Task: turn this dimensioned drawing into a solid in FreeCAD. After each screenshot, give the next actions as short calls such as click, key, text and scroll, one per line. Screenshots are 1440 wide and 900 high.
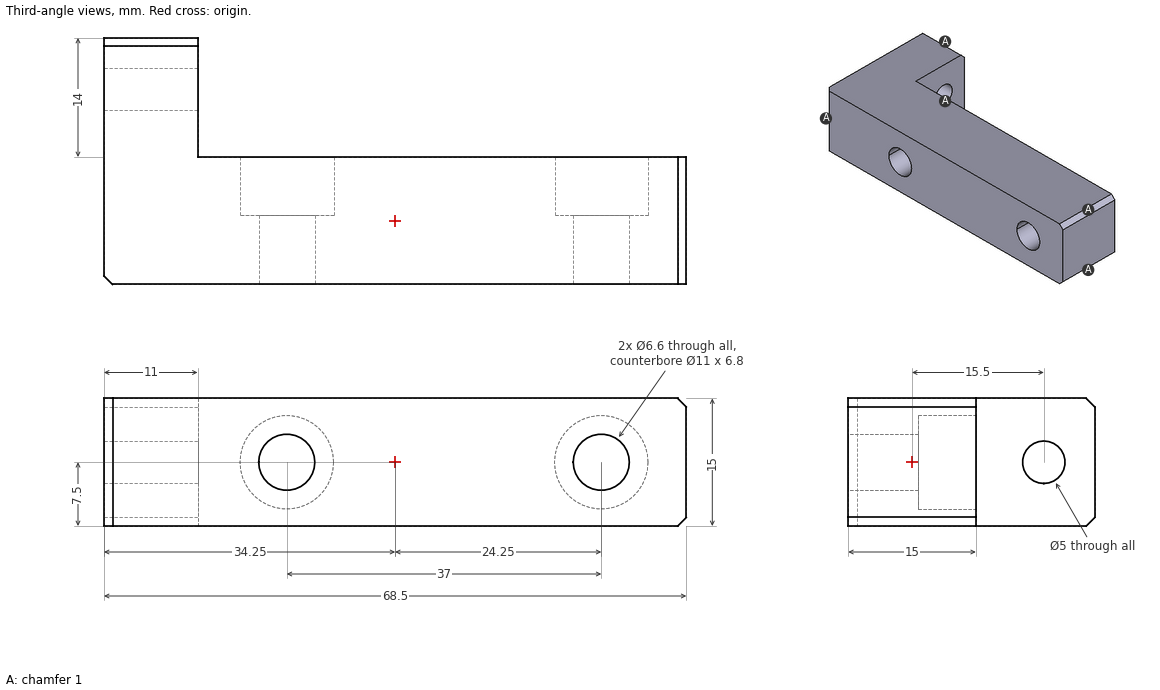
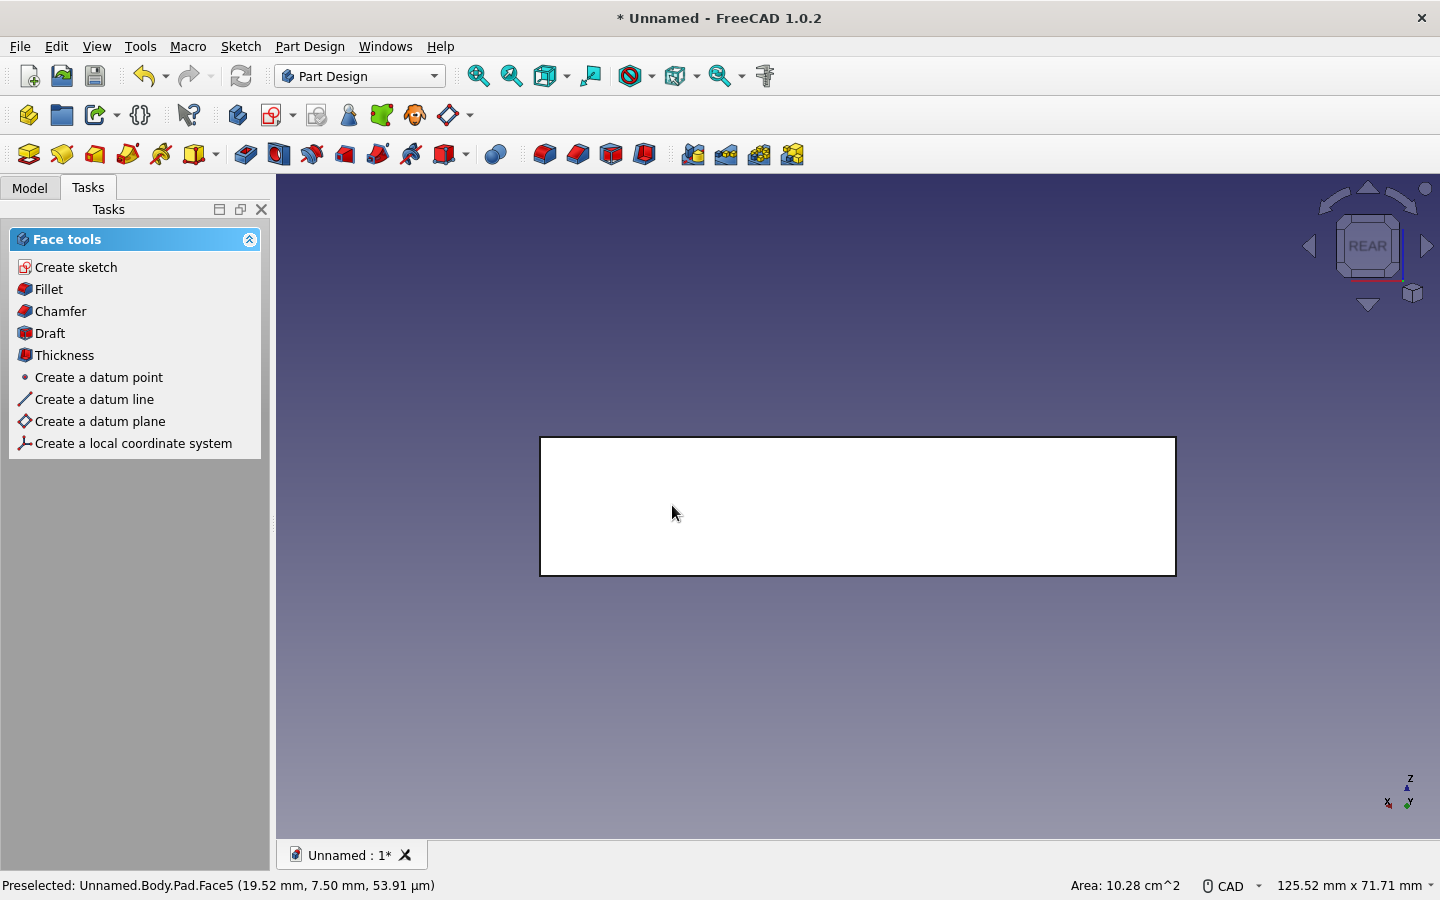
click(270, 116)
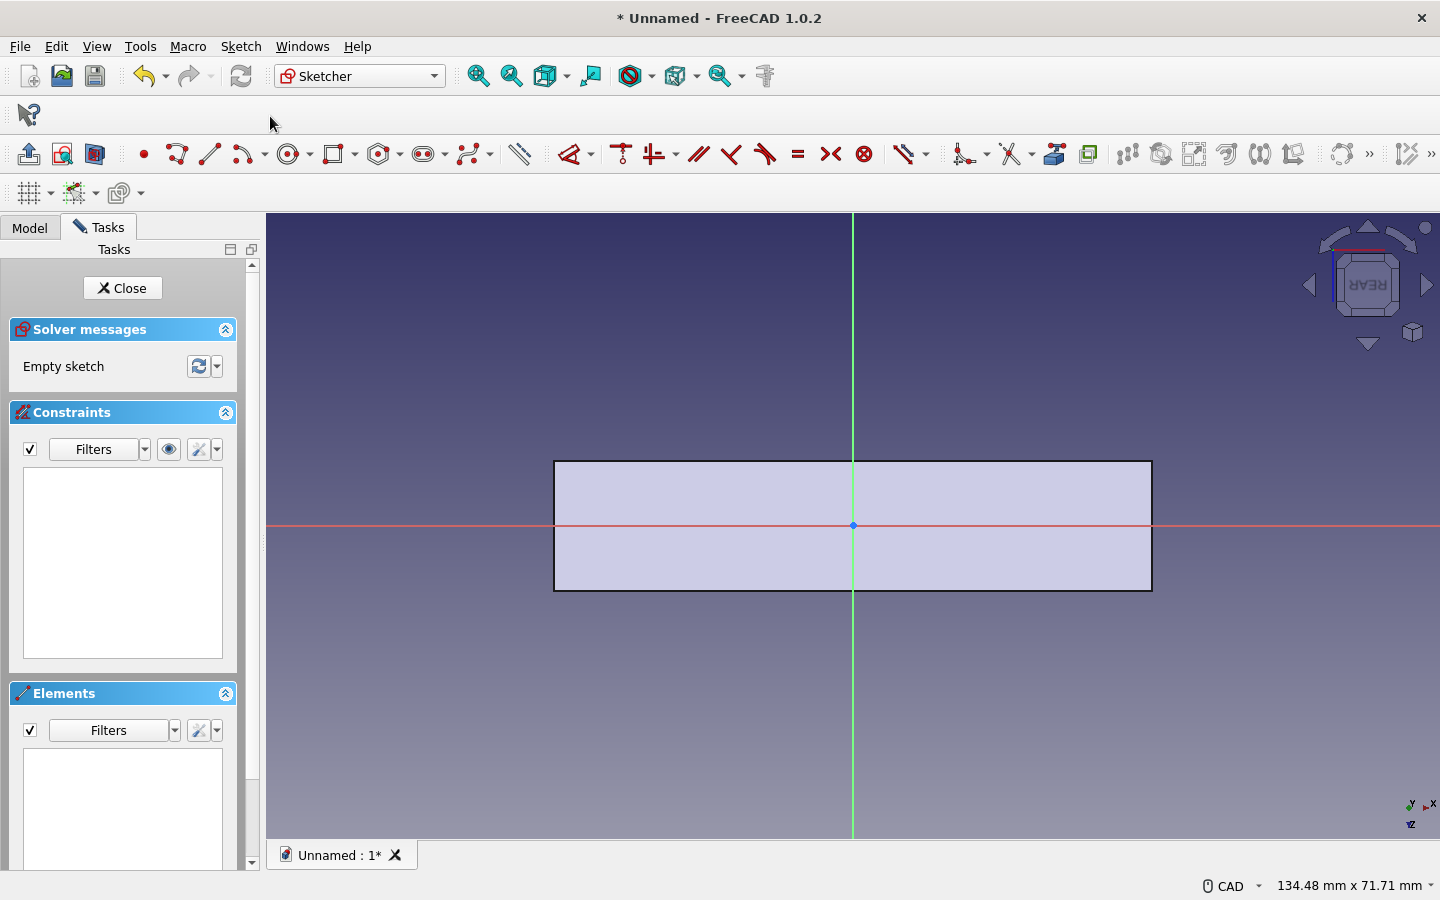
scroll(637, 526, up, 4)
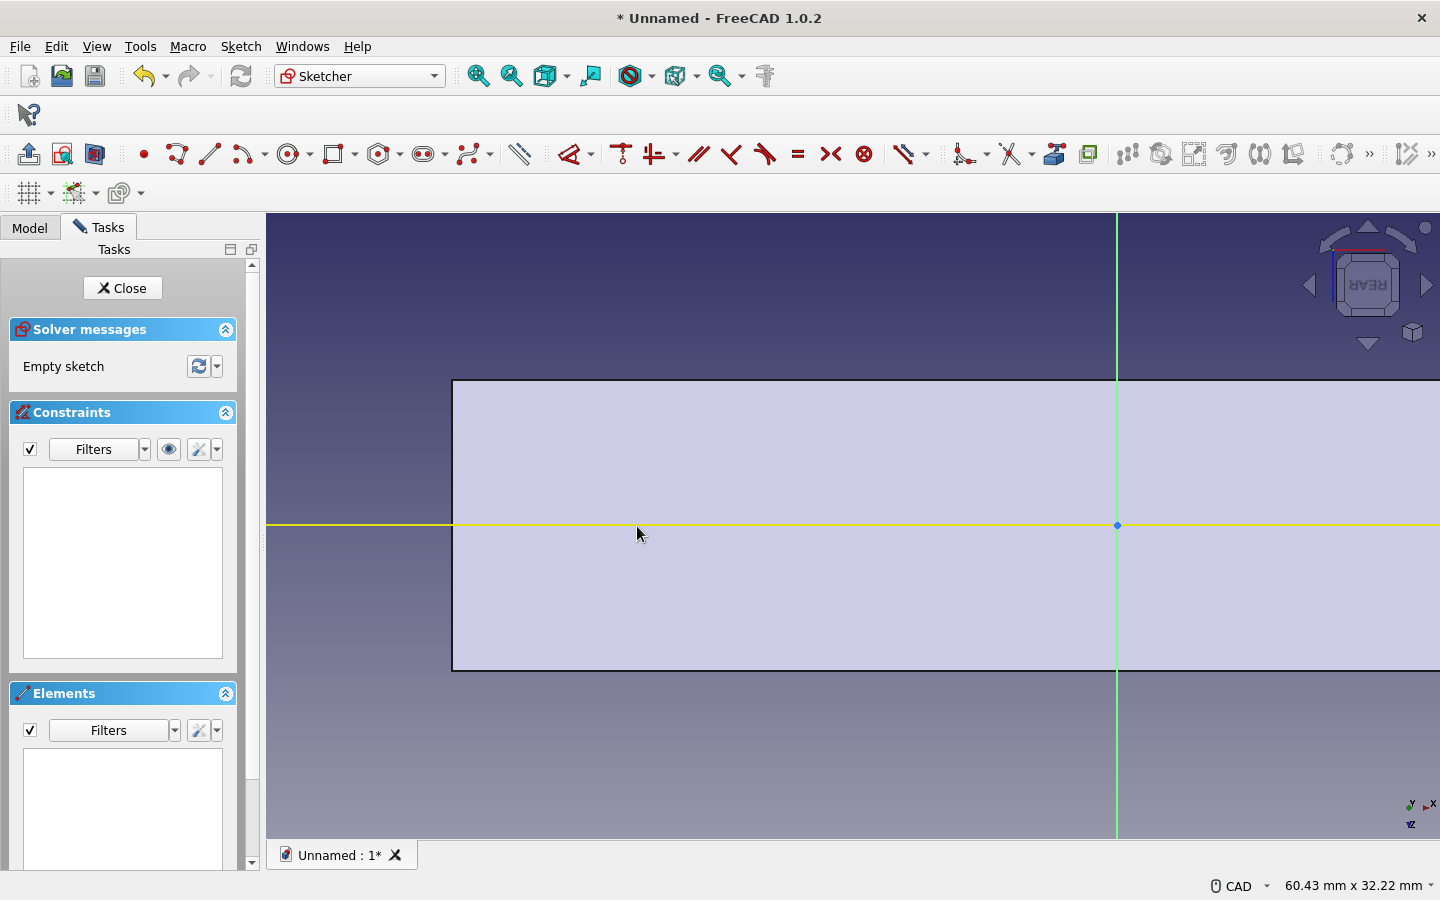
click(332, 154)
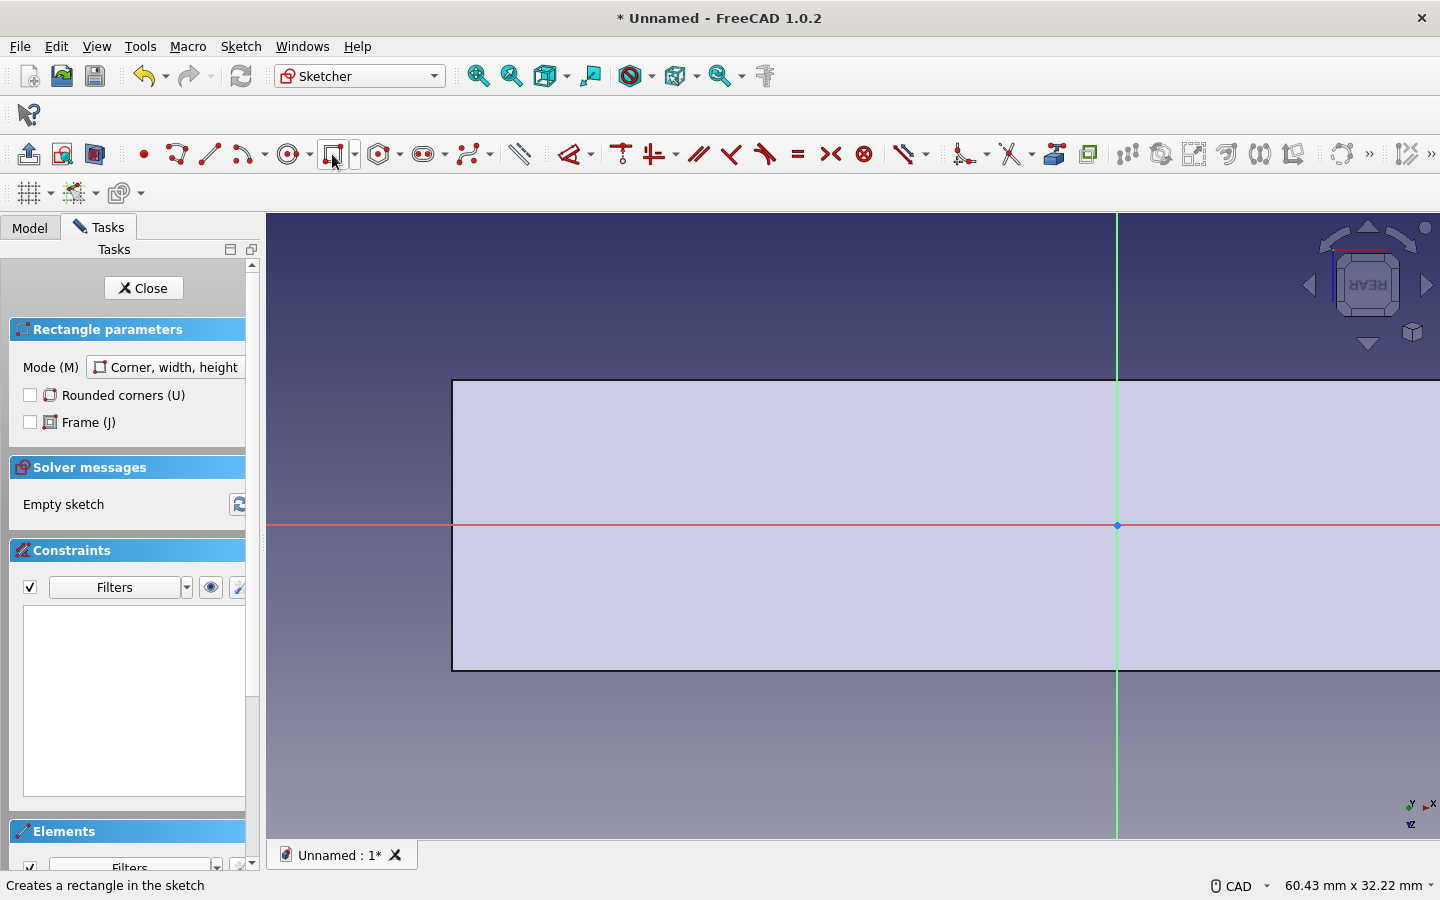
click(452, 380)
move(666, 671)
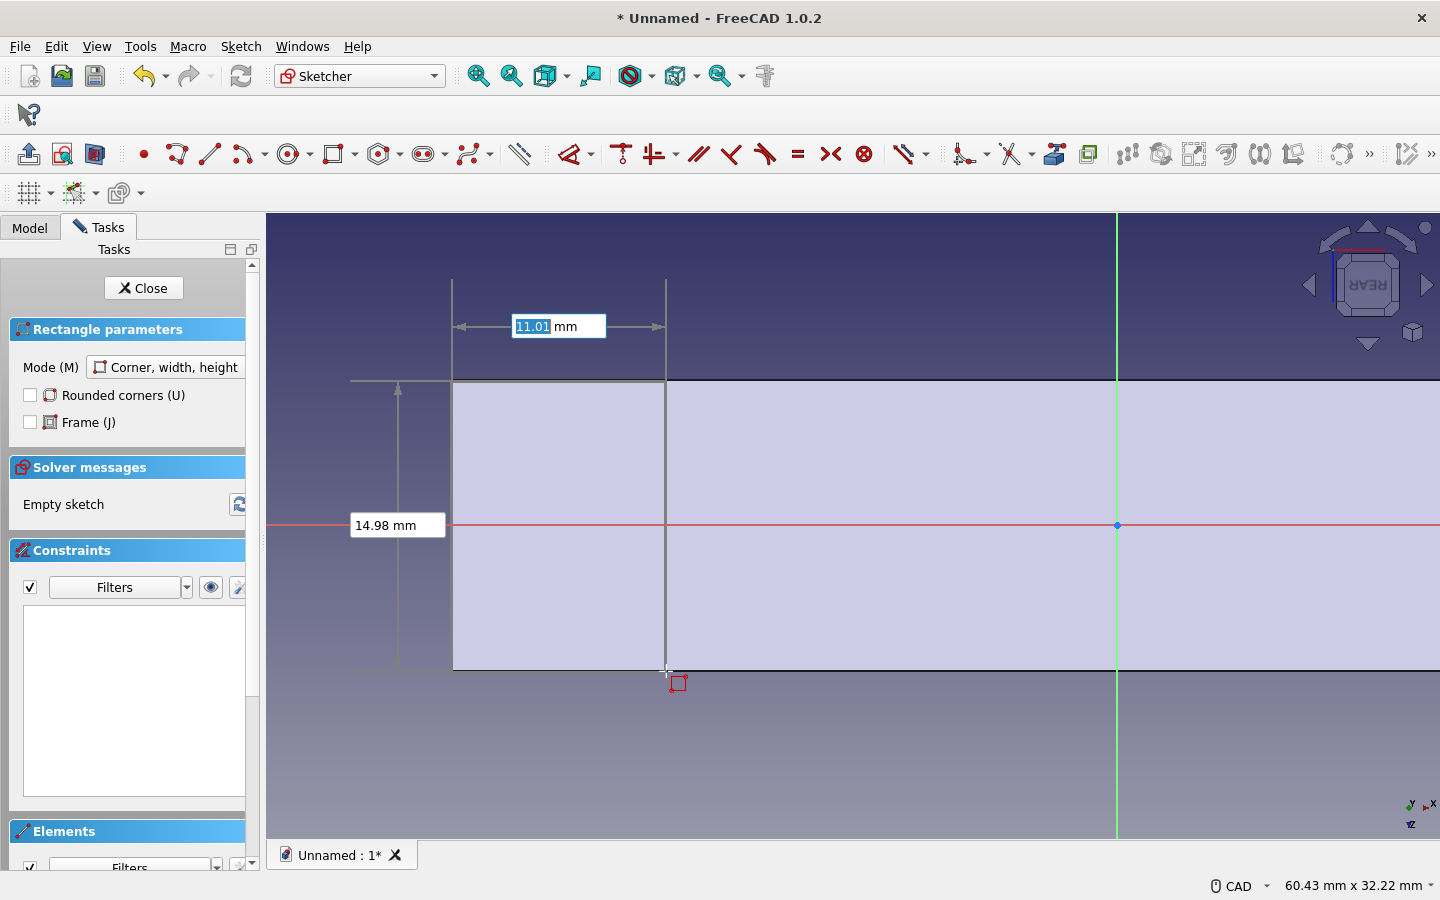
text(11)
key(Tab)
text(15)
key(Return)
key(Escape)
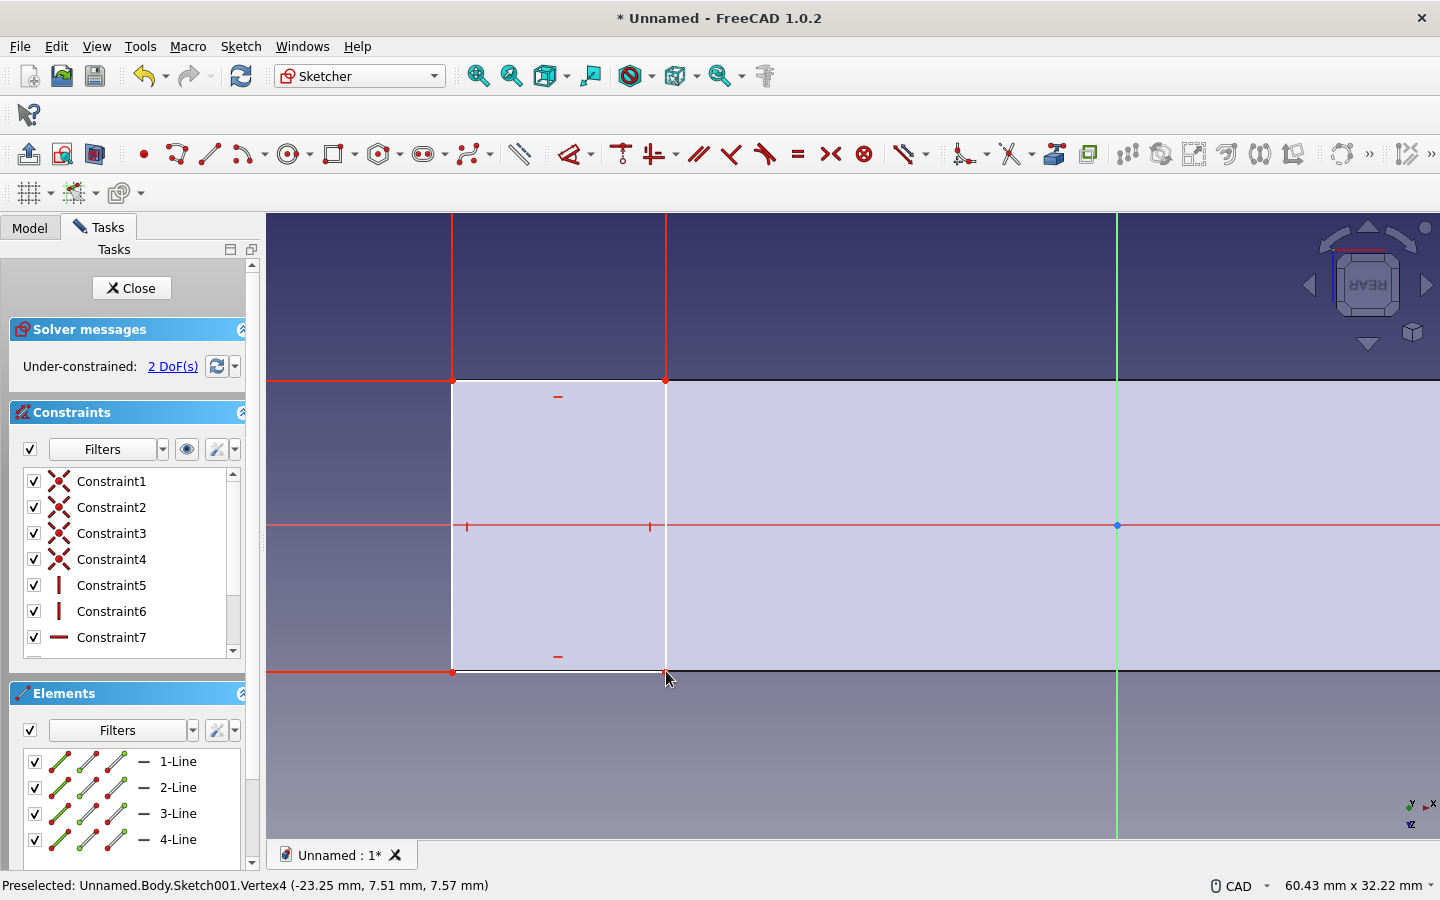
click(568, 154)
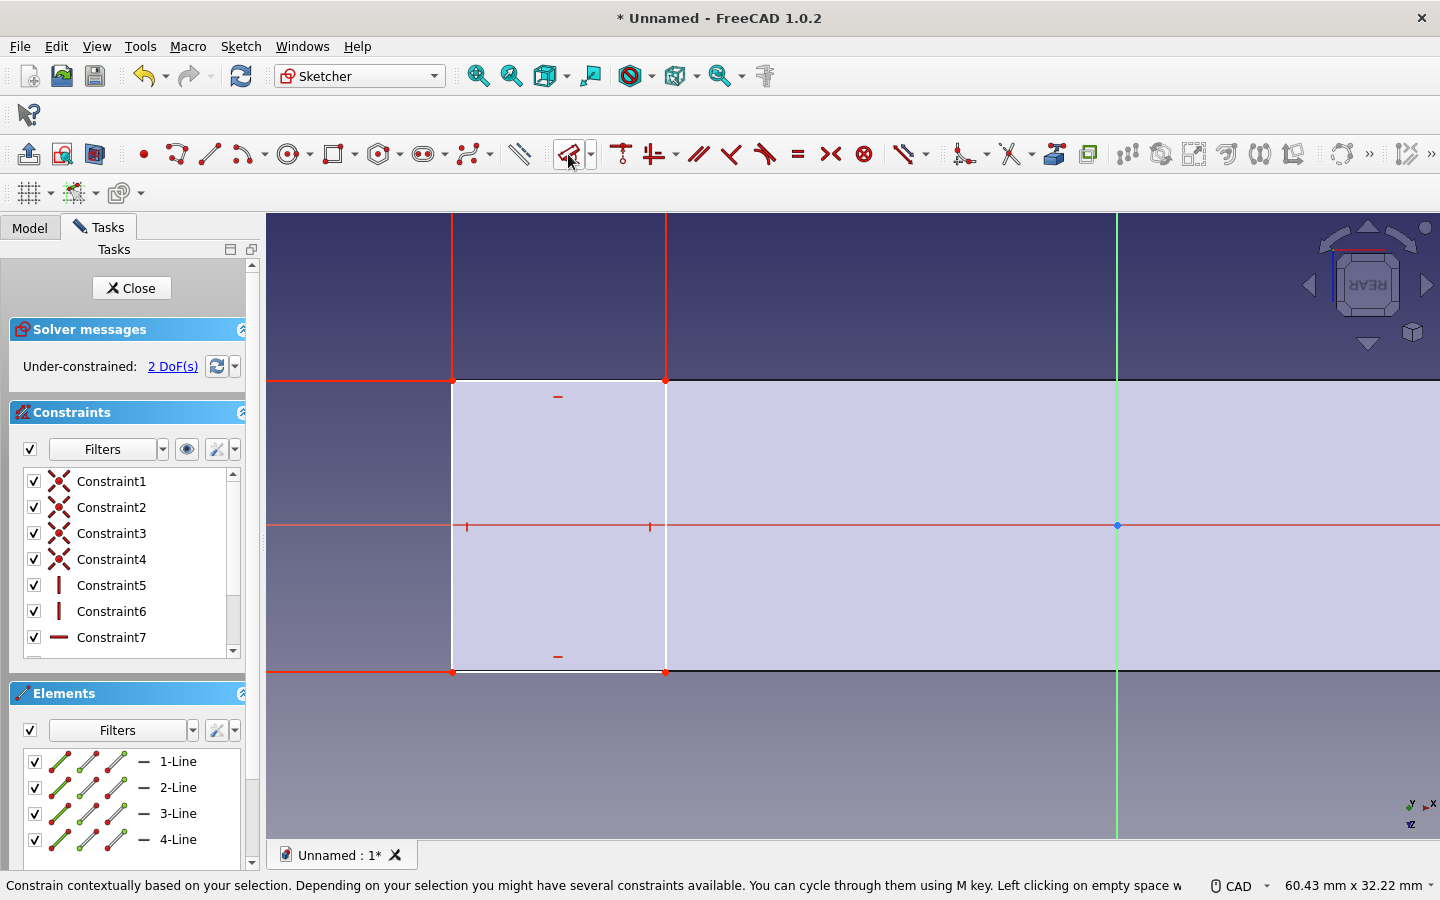
click(452, 381)
click(1151, 453)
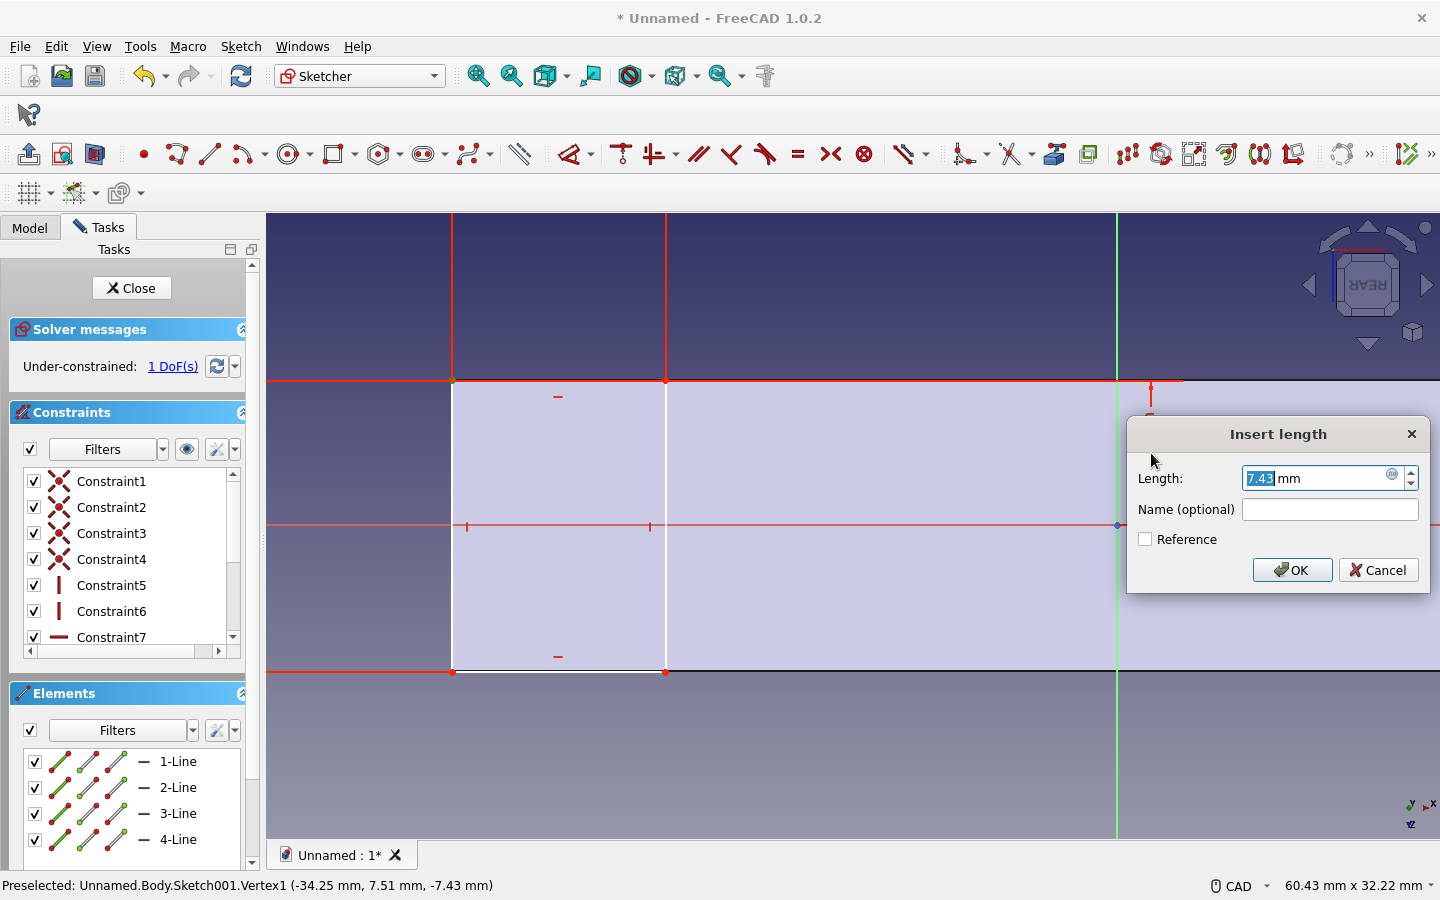
text(7.5)
key(Return)